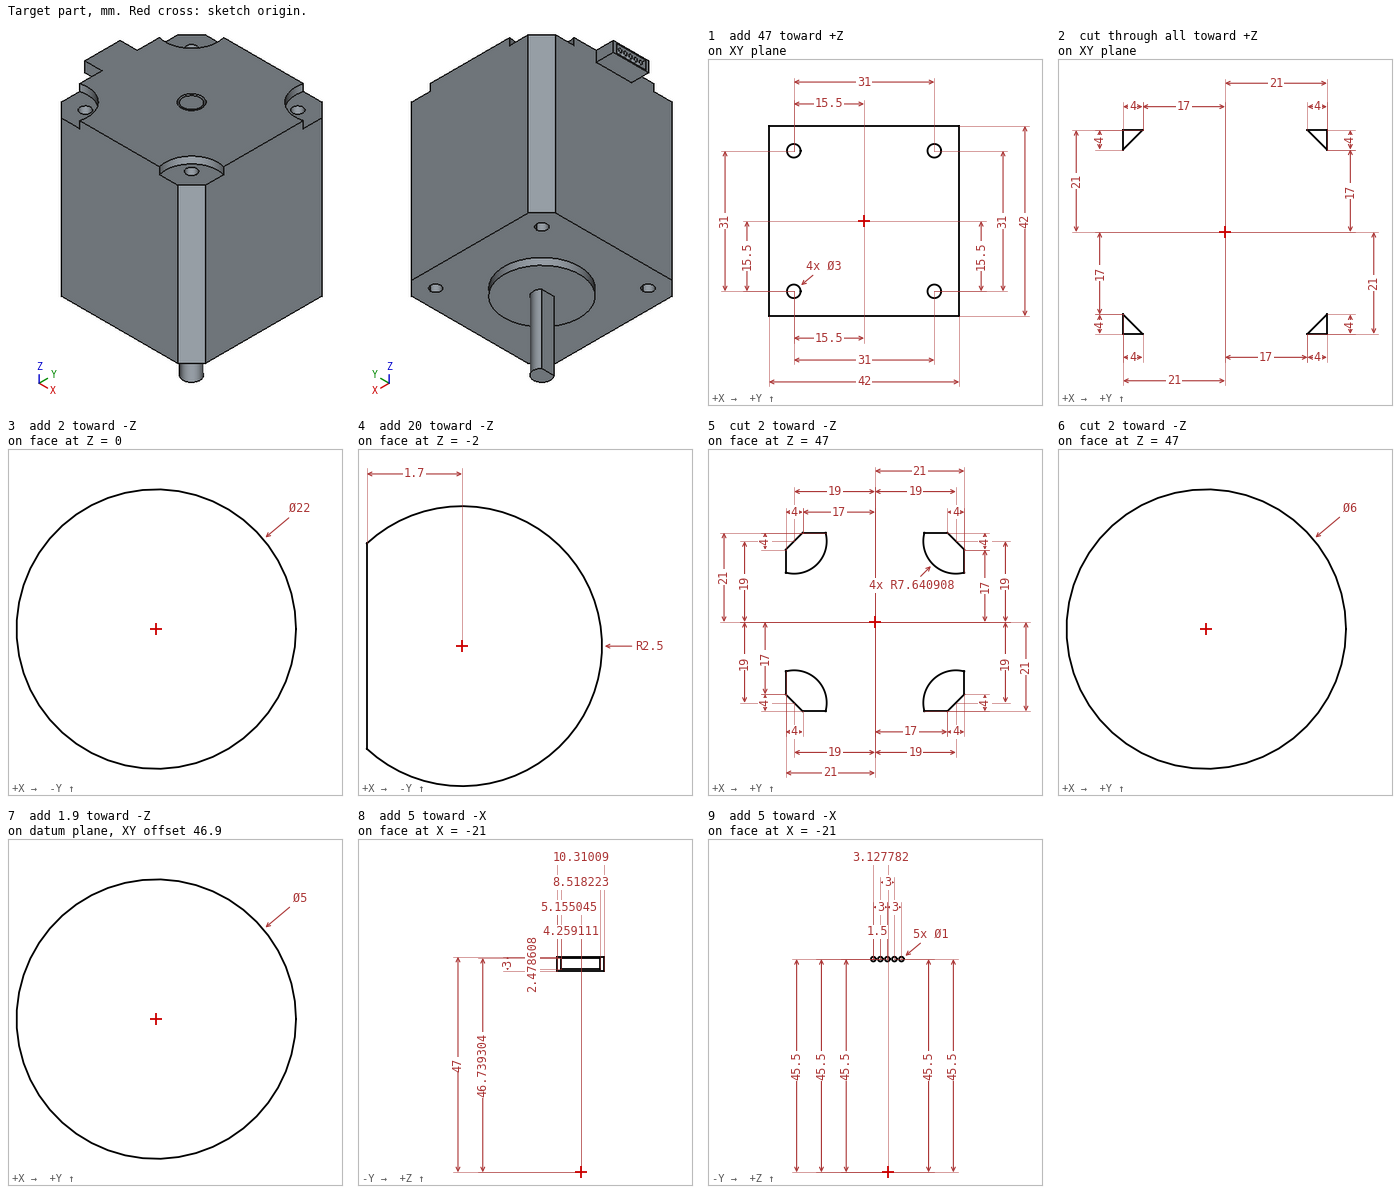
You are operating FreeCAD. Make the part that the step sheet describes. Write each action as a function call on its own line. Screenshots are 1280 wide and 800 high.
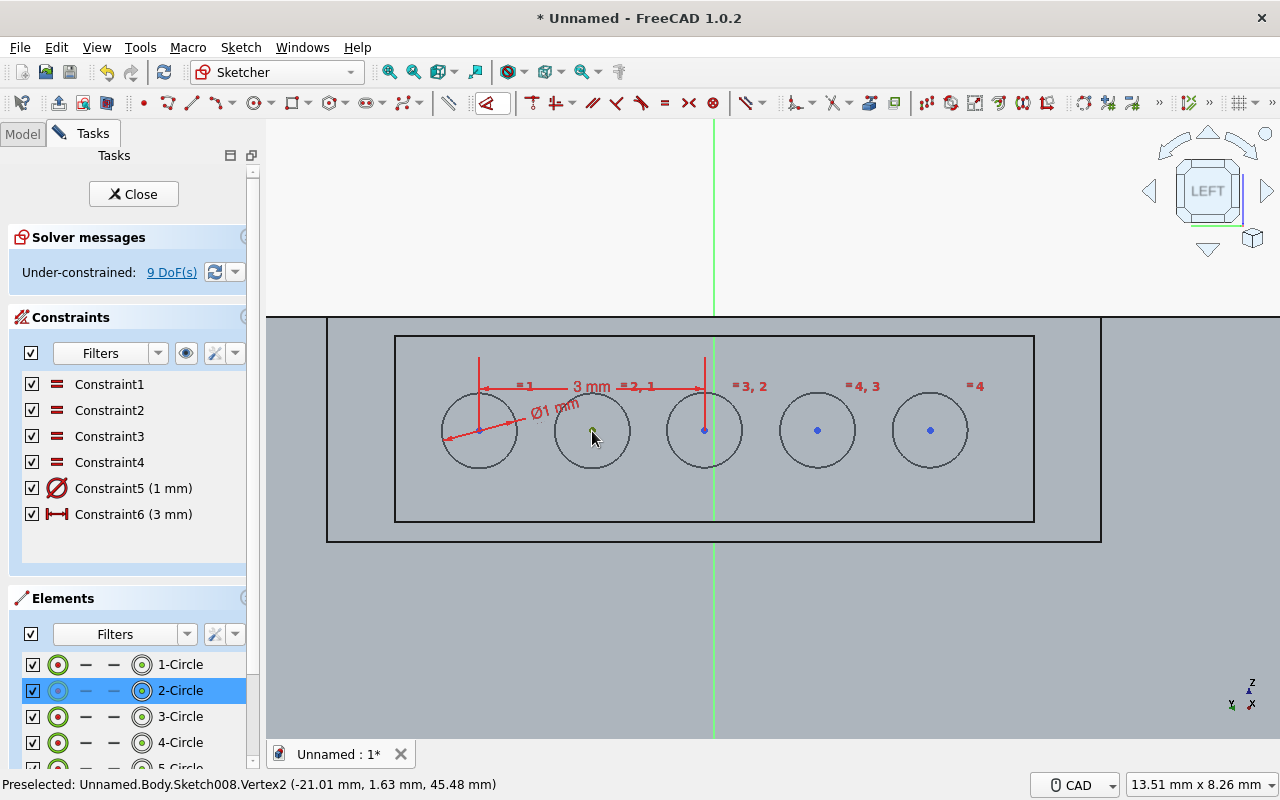
click(818, 430)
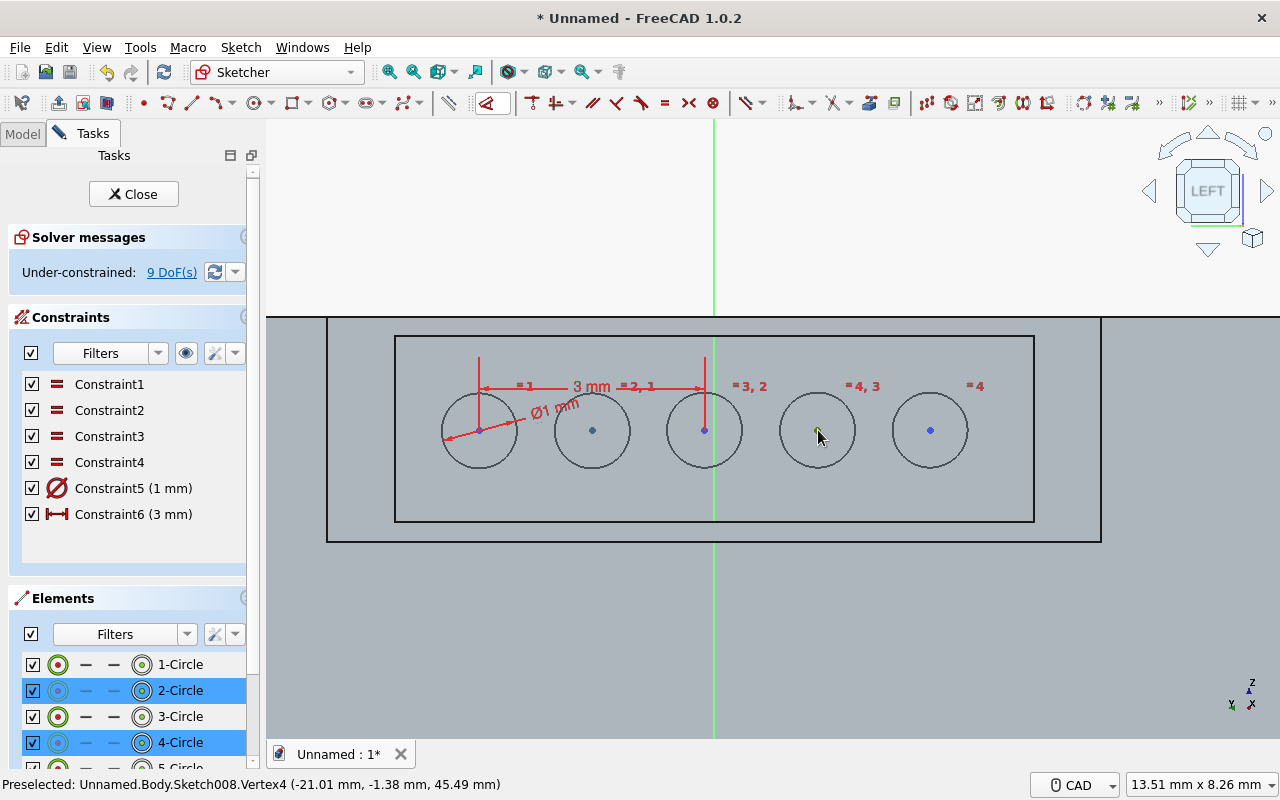
click(504, 104)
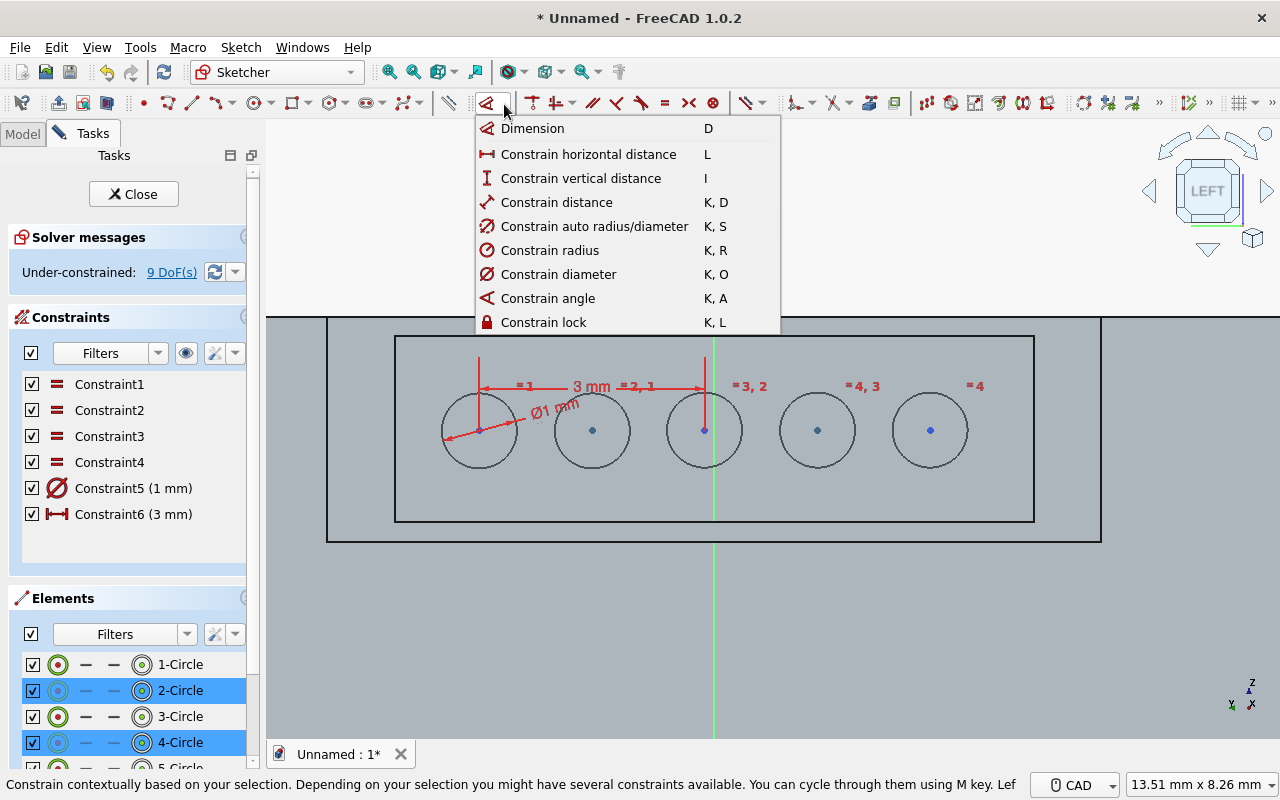
click(628, 154)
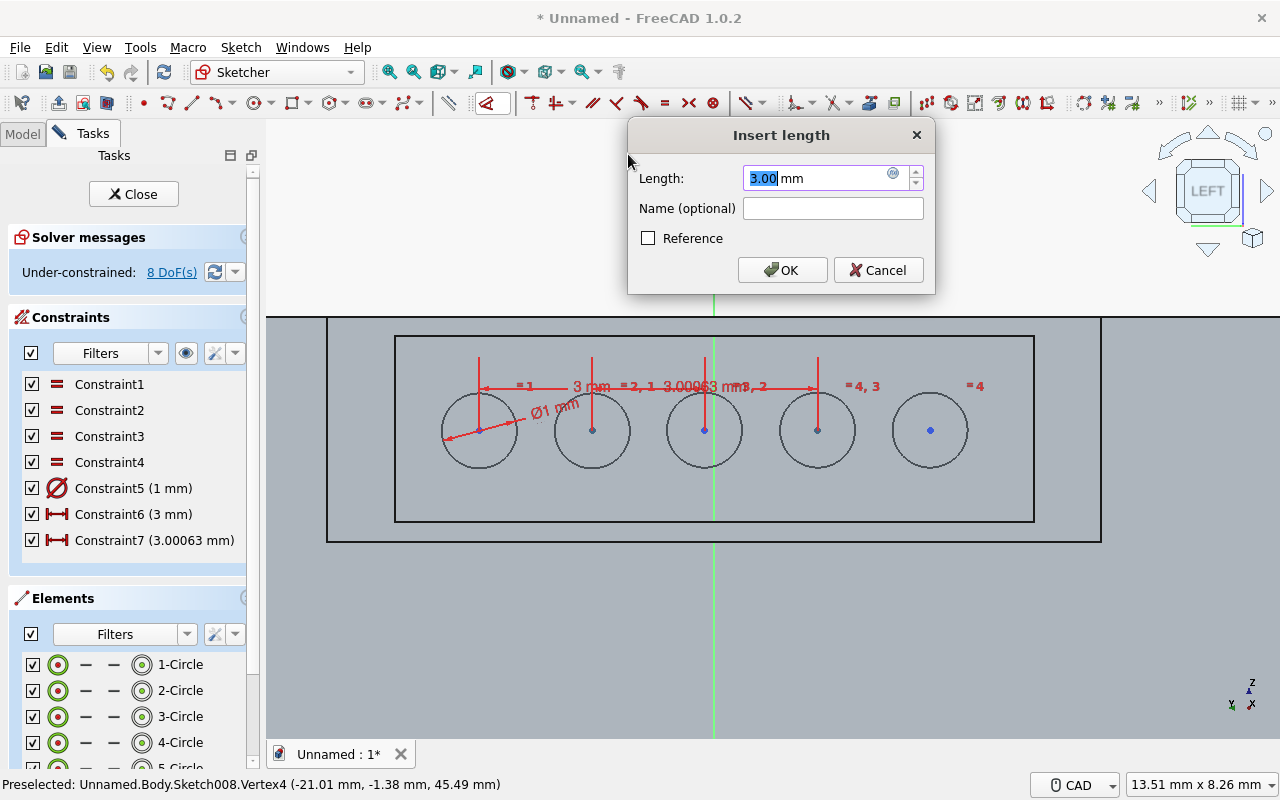
text(3)
key(Return)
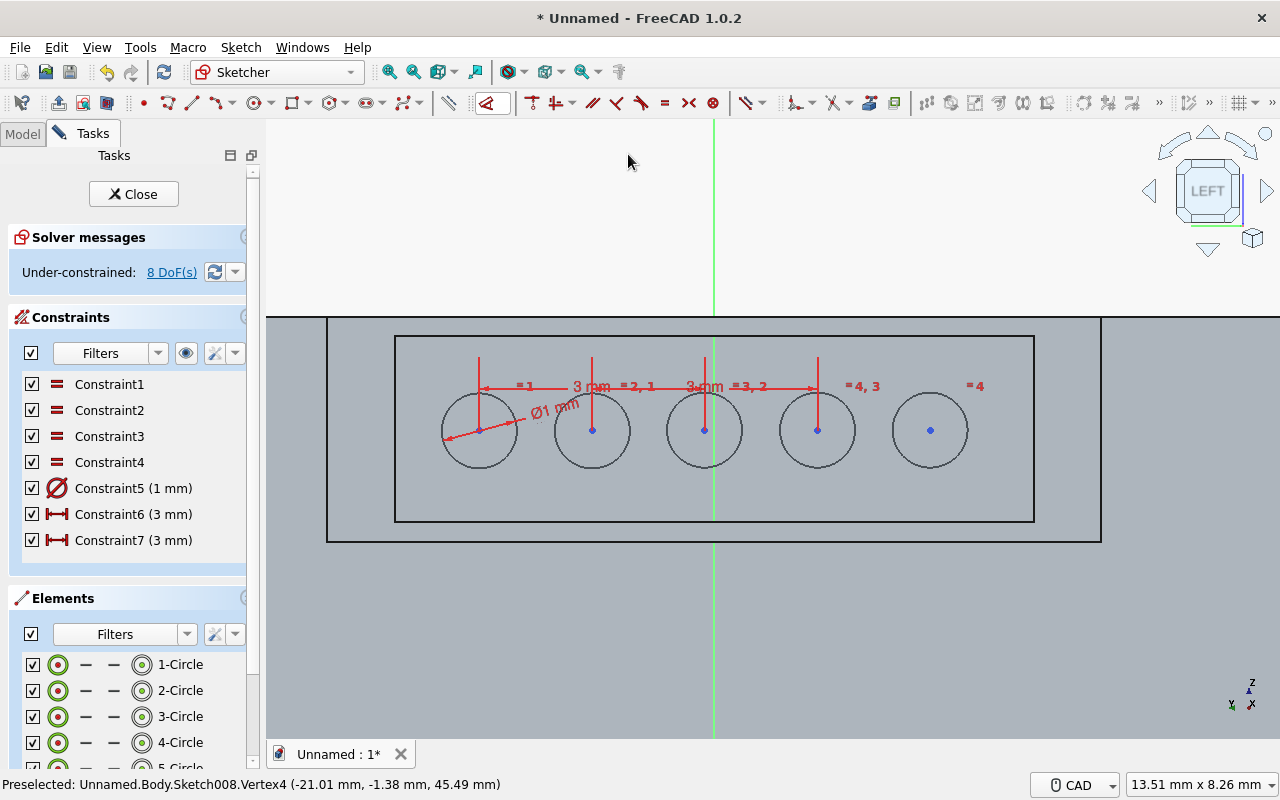
click(705, 430)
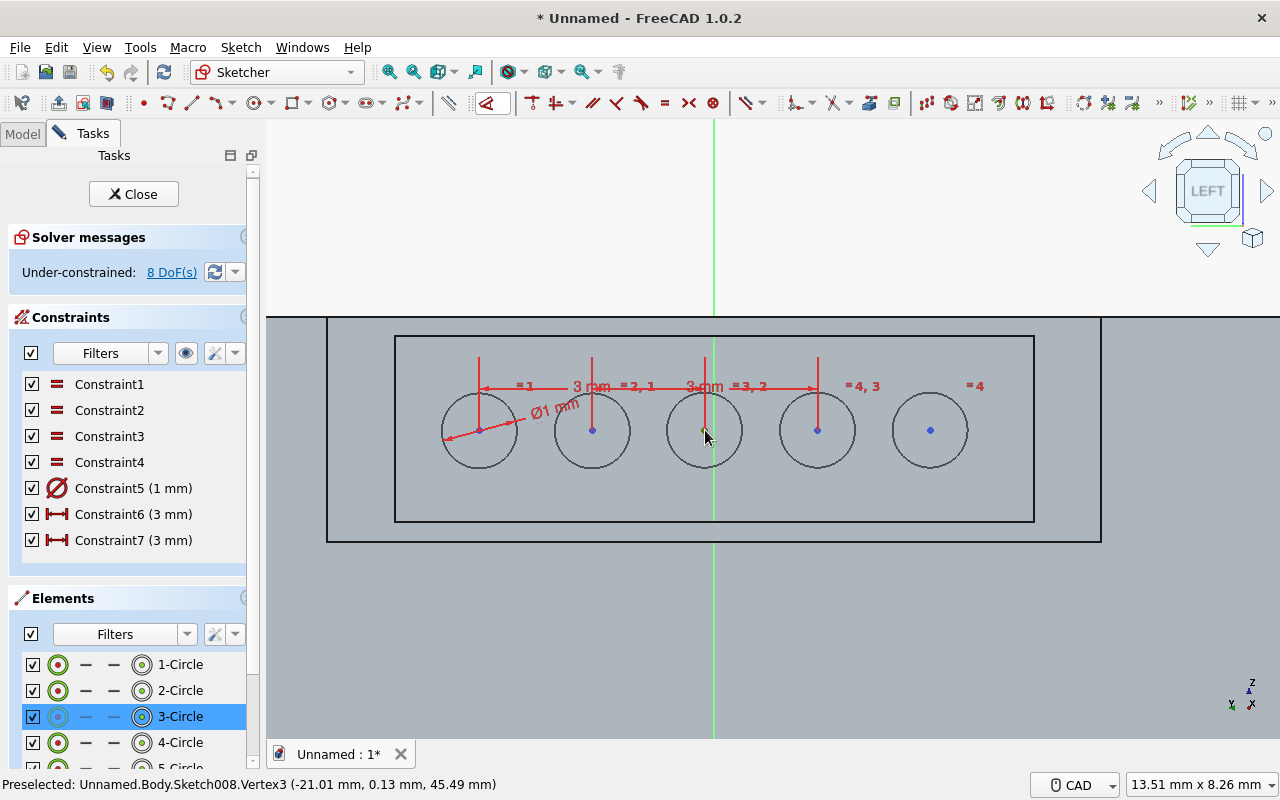
click(930, 430)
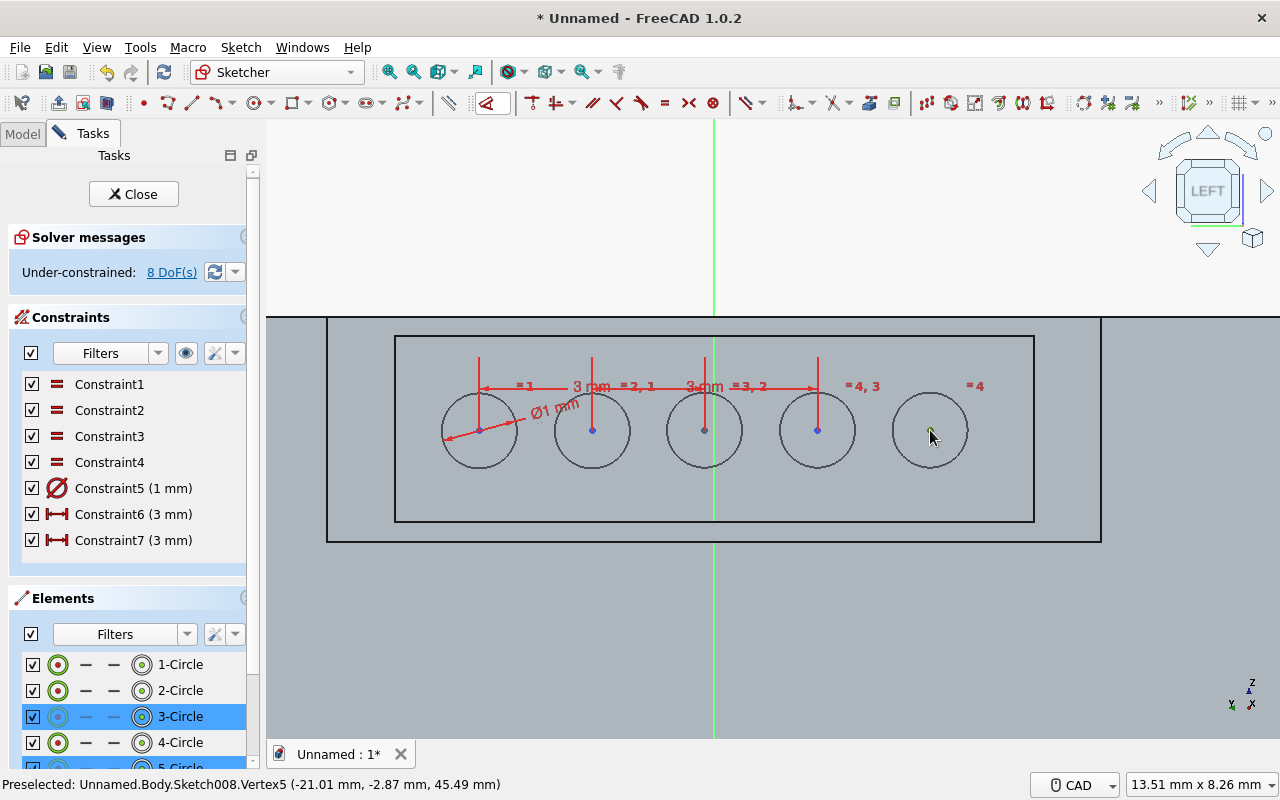
key(l)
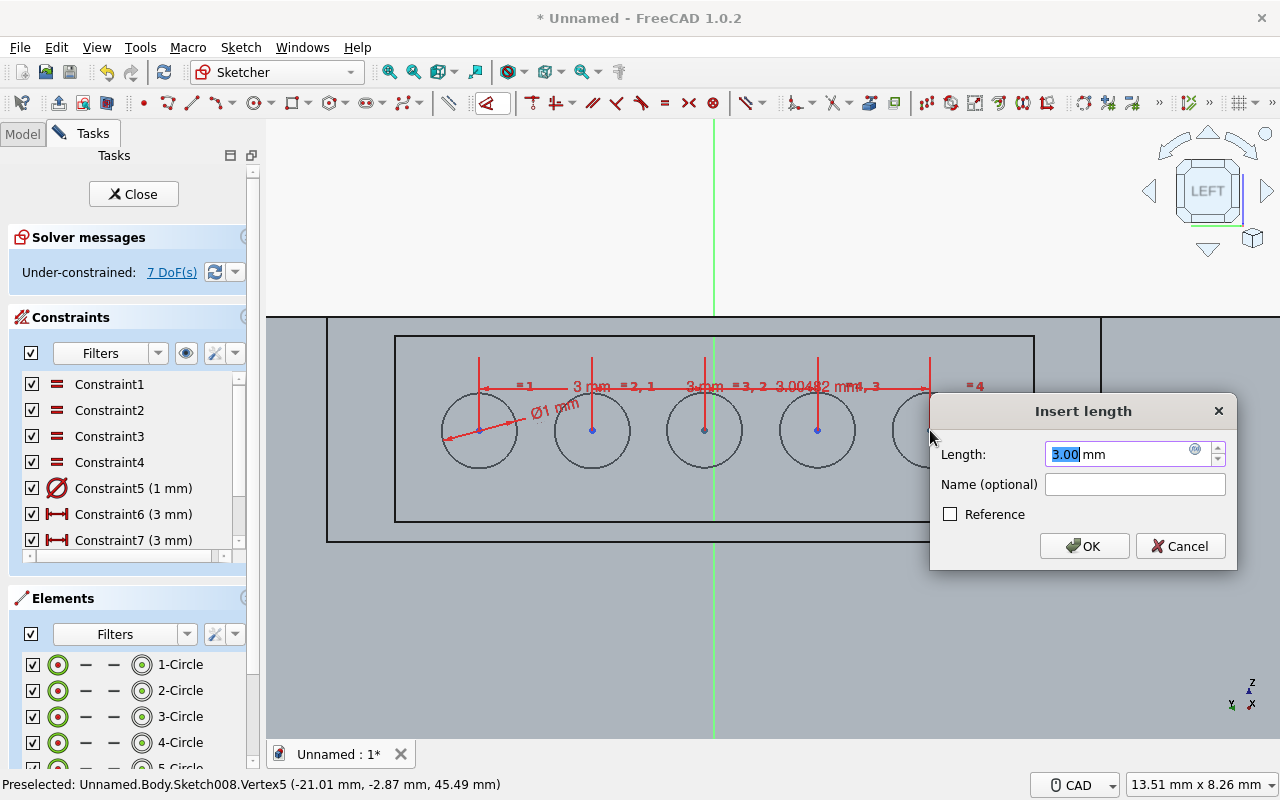
text(3)
key(Return)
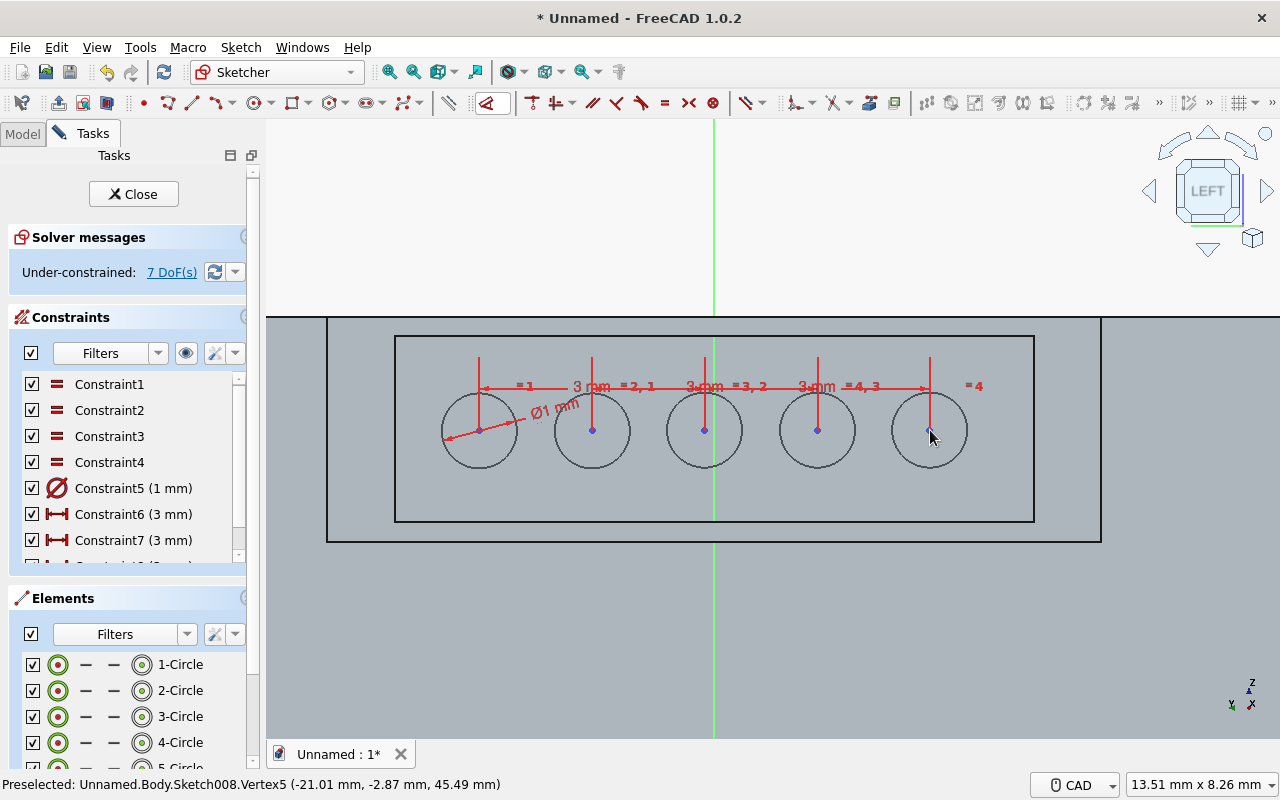
click(479, 431)